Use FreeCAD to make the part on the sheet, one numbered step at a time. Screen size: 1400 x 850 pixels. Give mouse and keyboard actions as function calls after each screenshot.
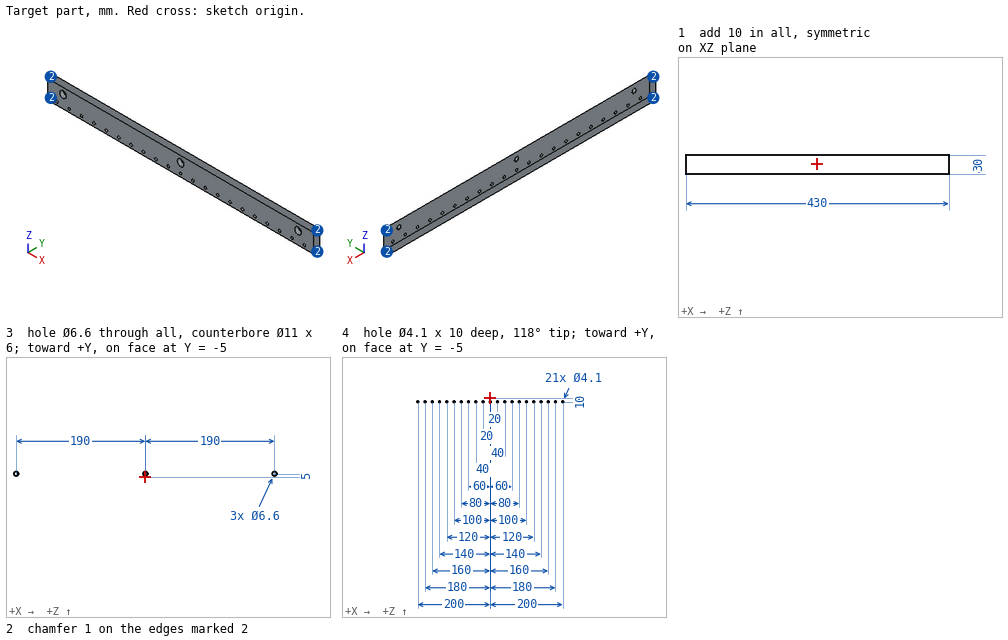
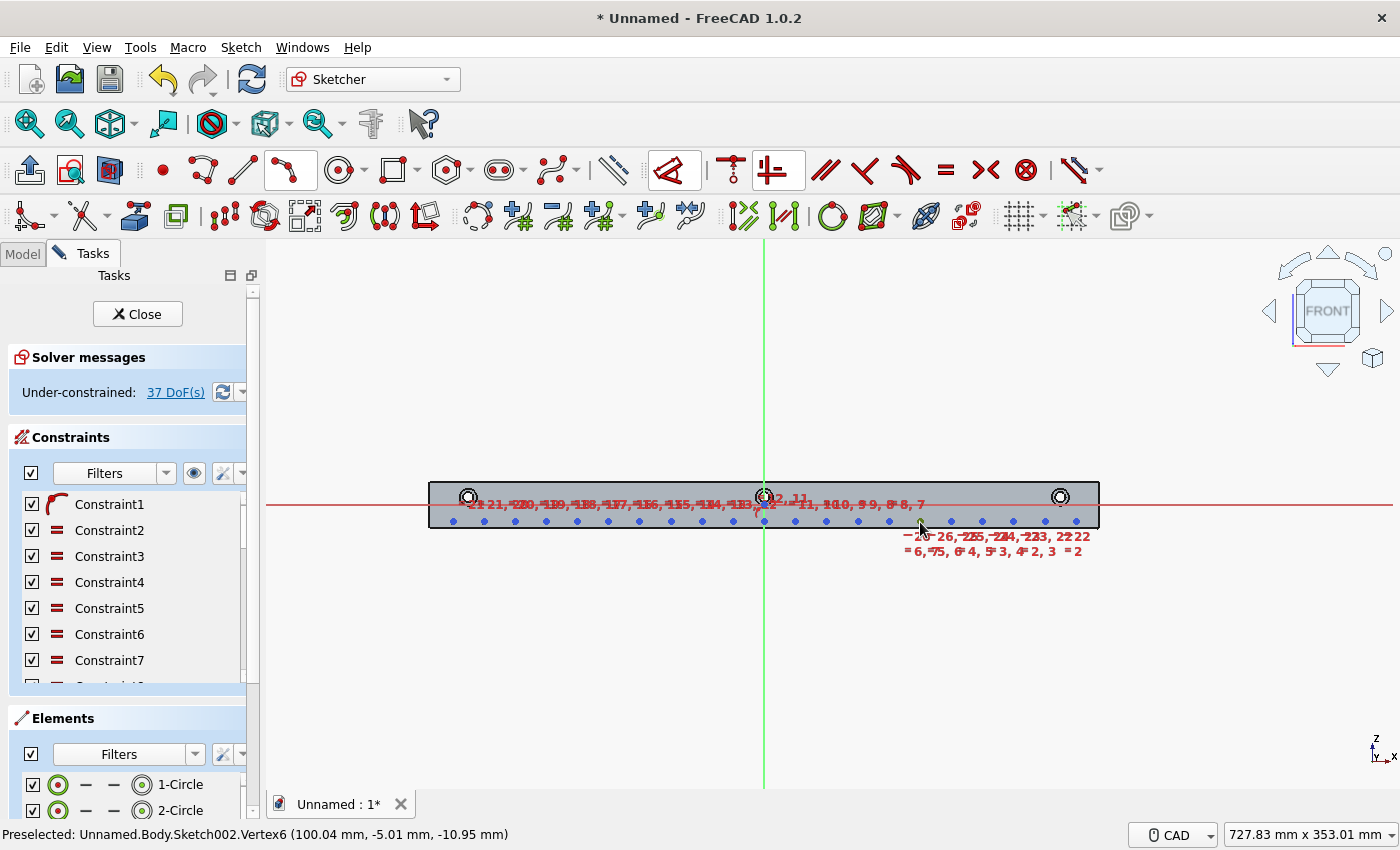
click(889, 522)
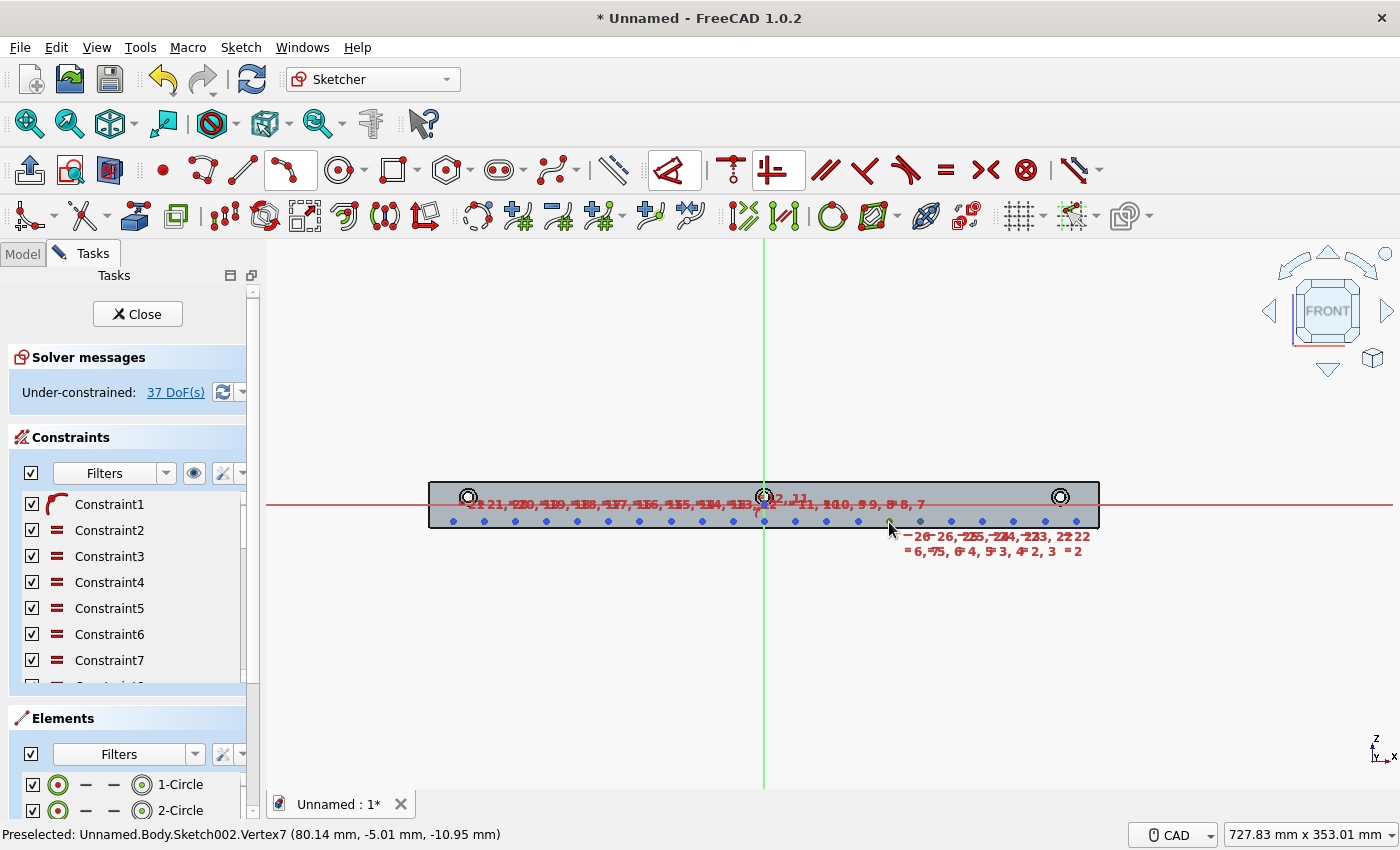
click(800, 170)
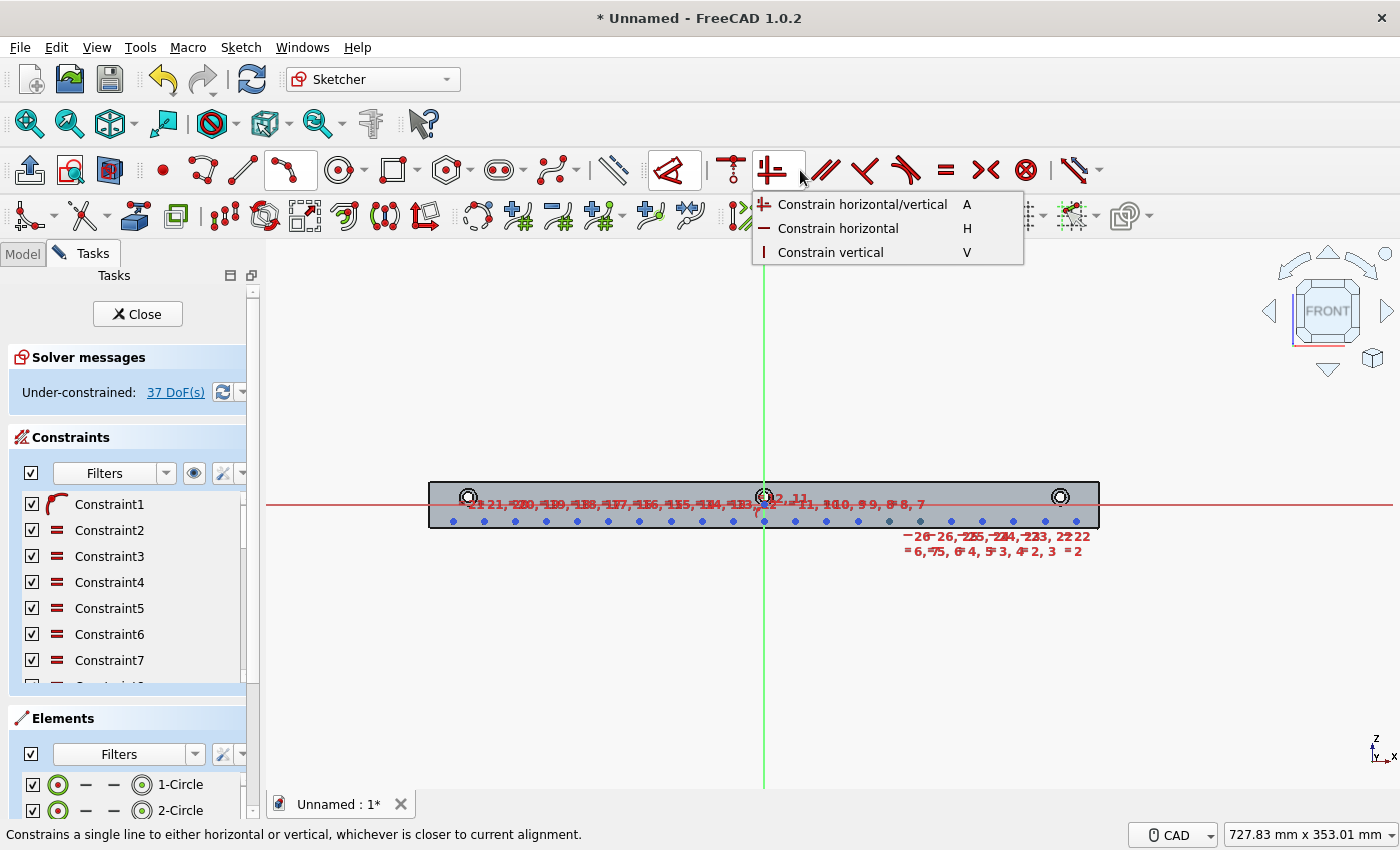
click(888, 228)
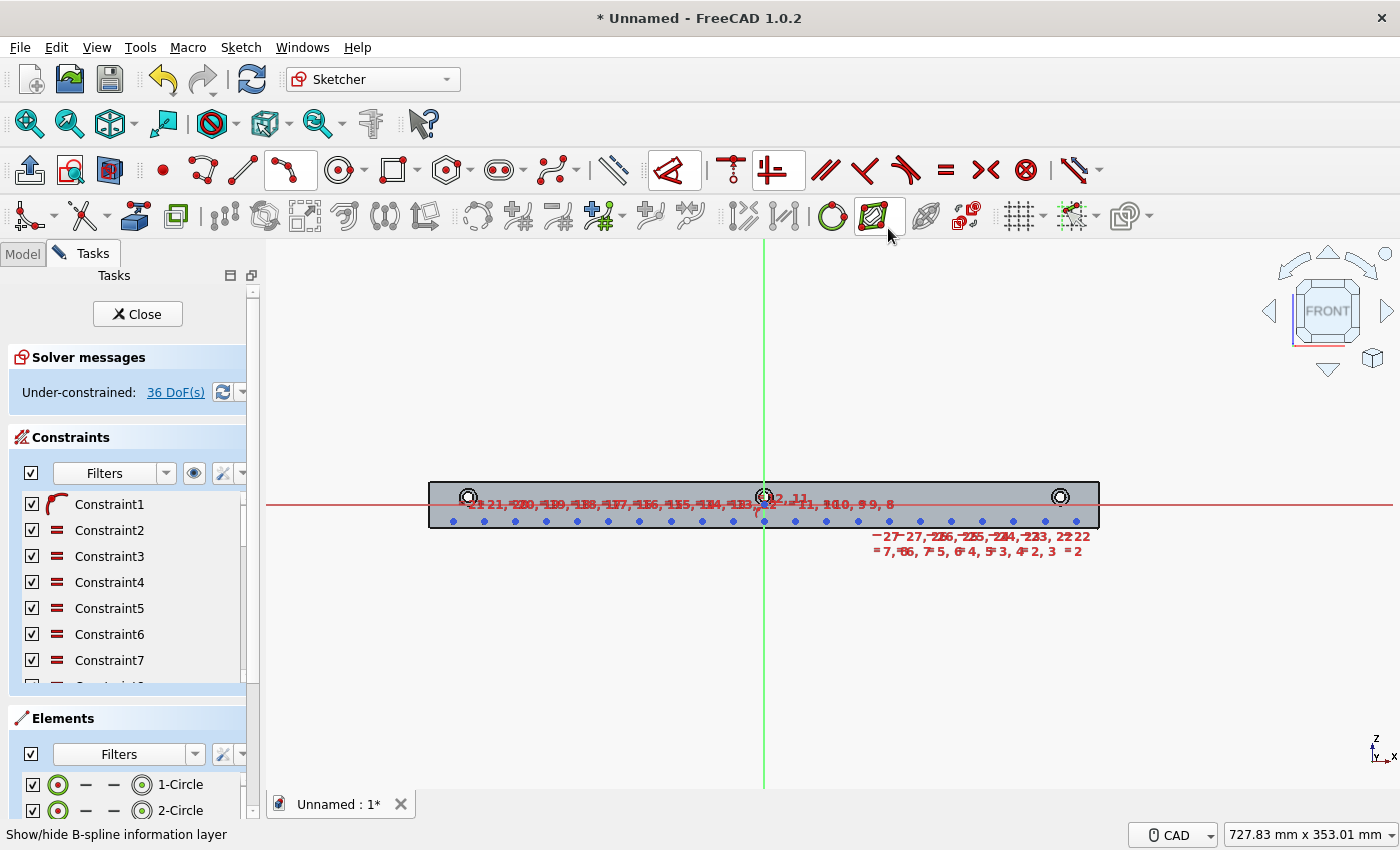
click(889, 522)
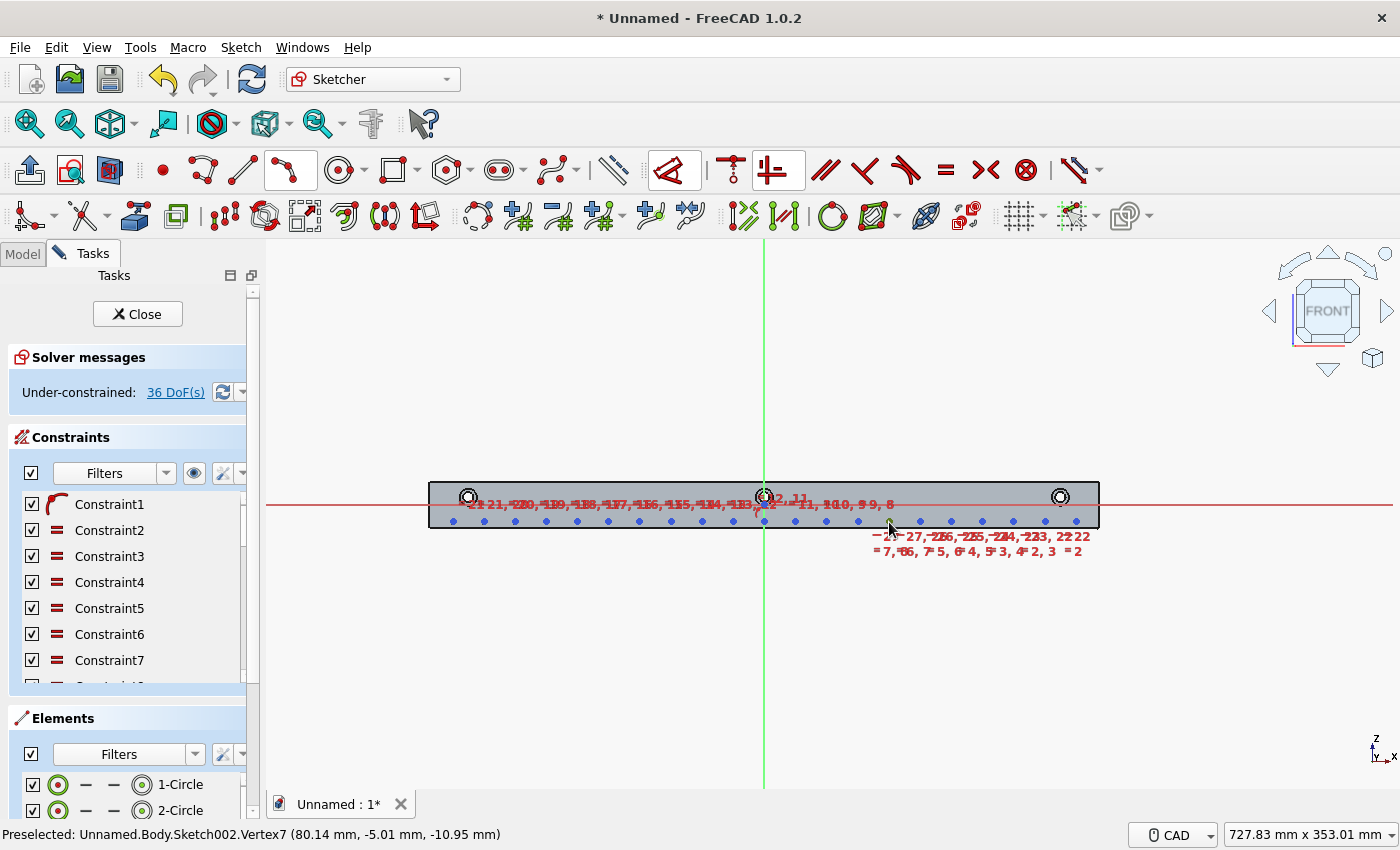
click(858, 522)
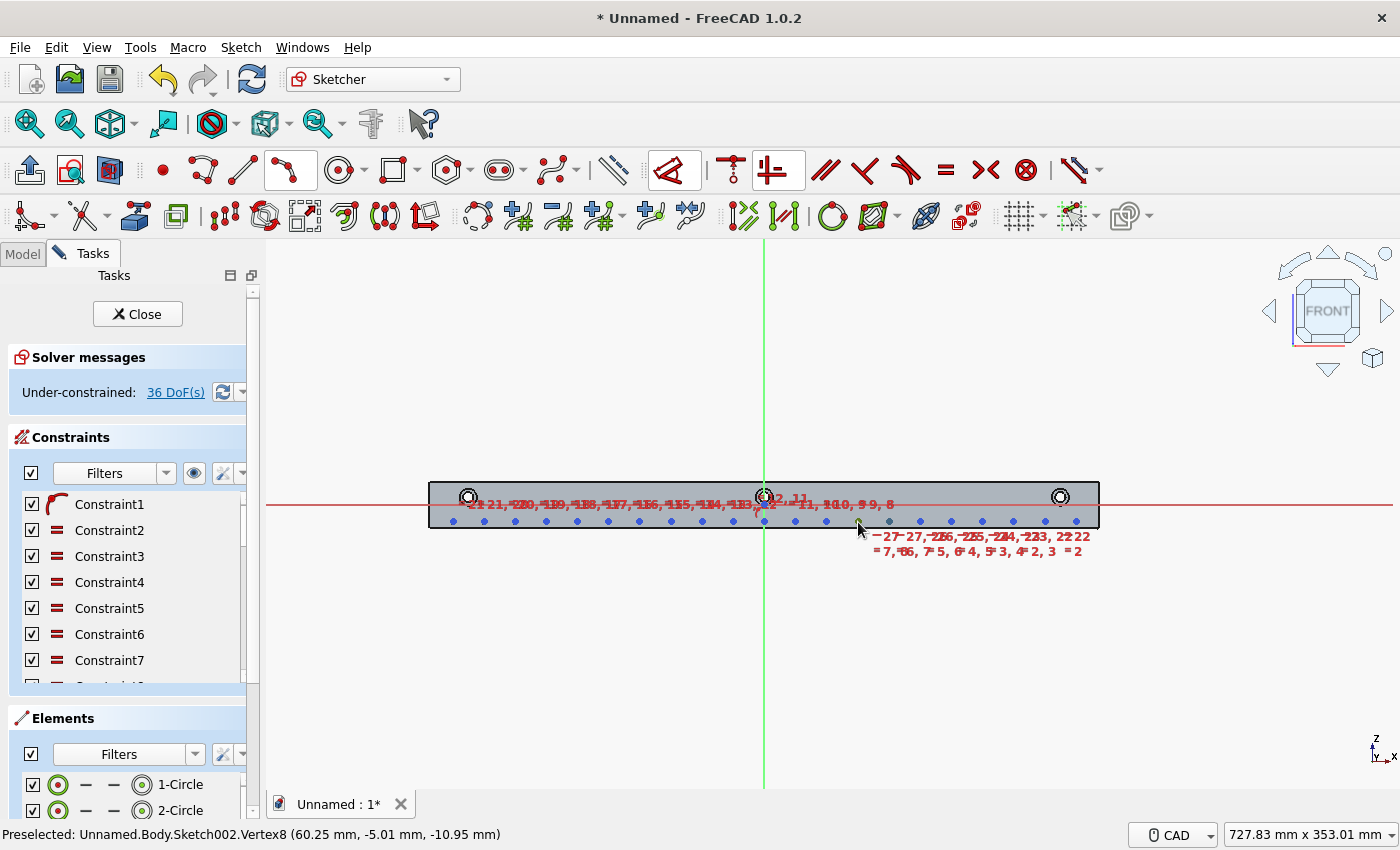
click(800, 170)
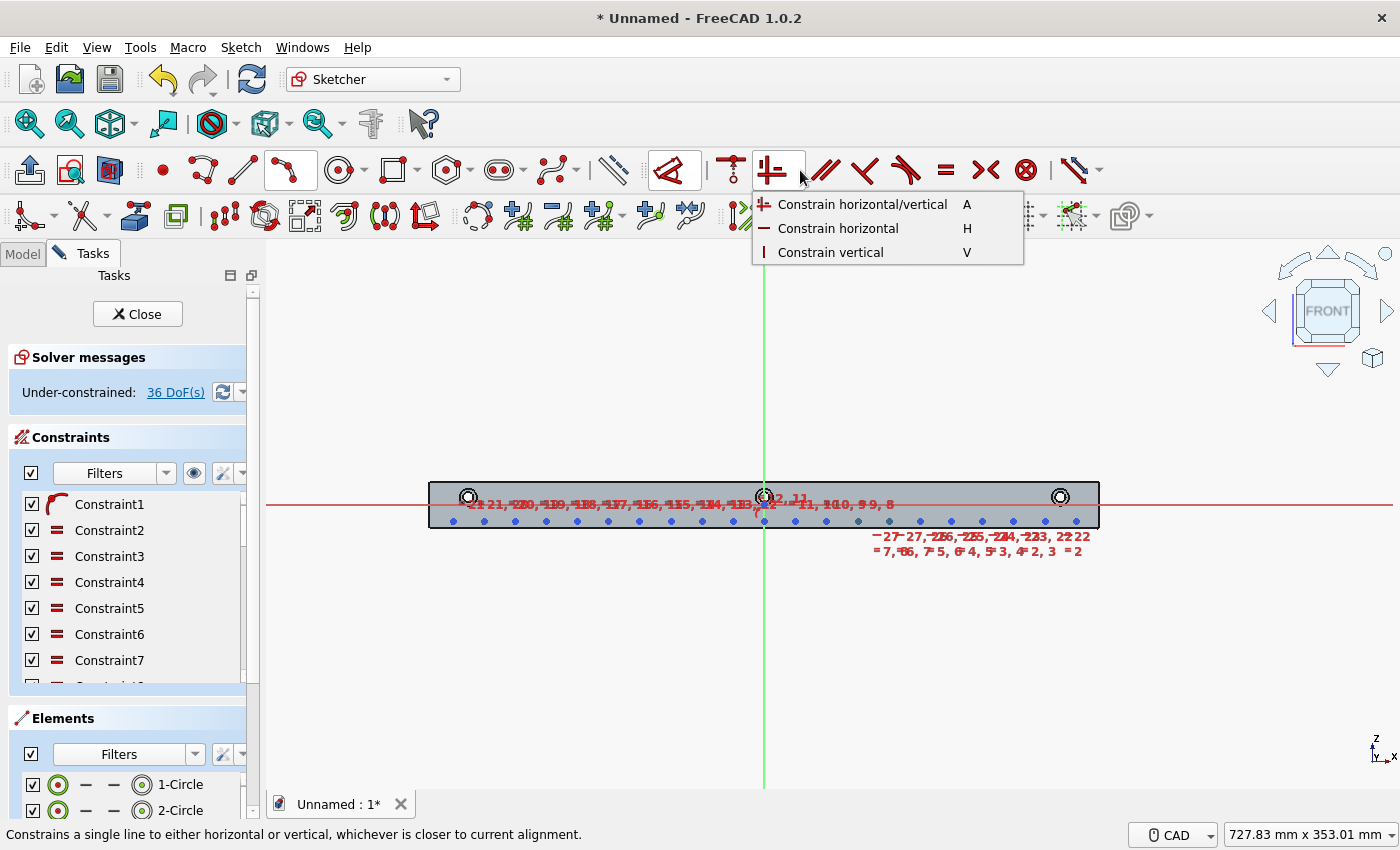
click(888, 228)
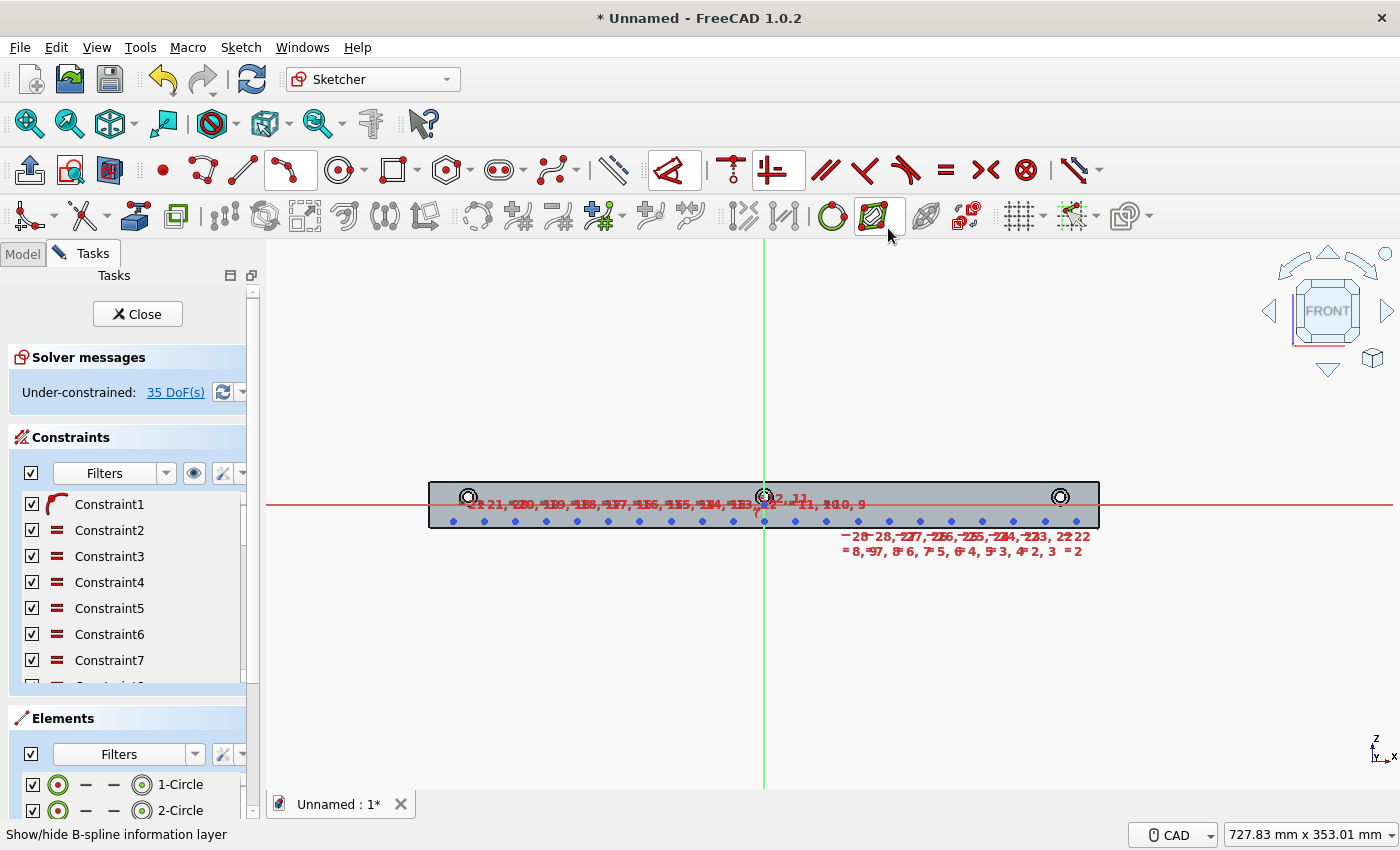
click(858, 522)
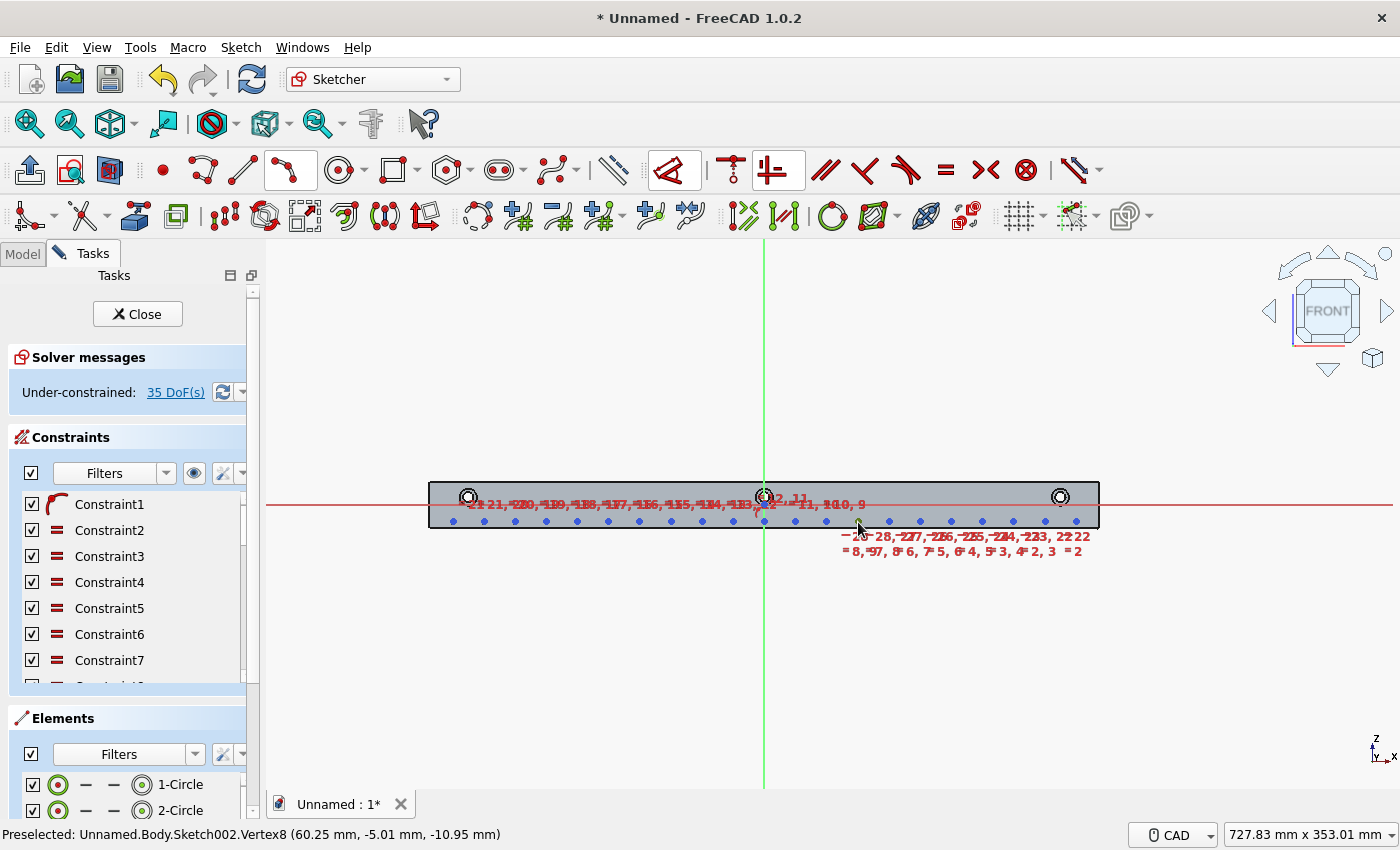
click(826, 522)